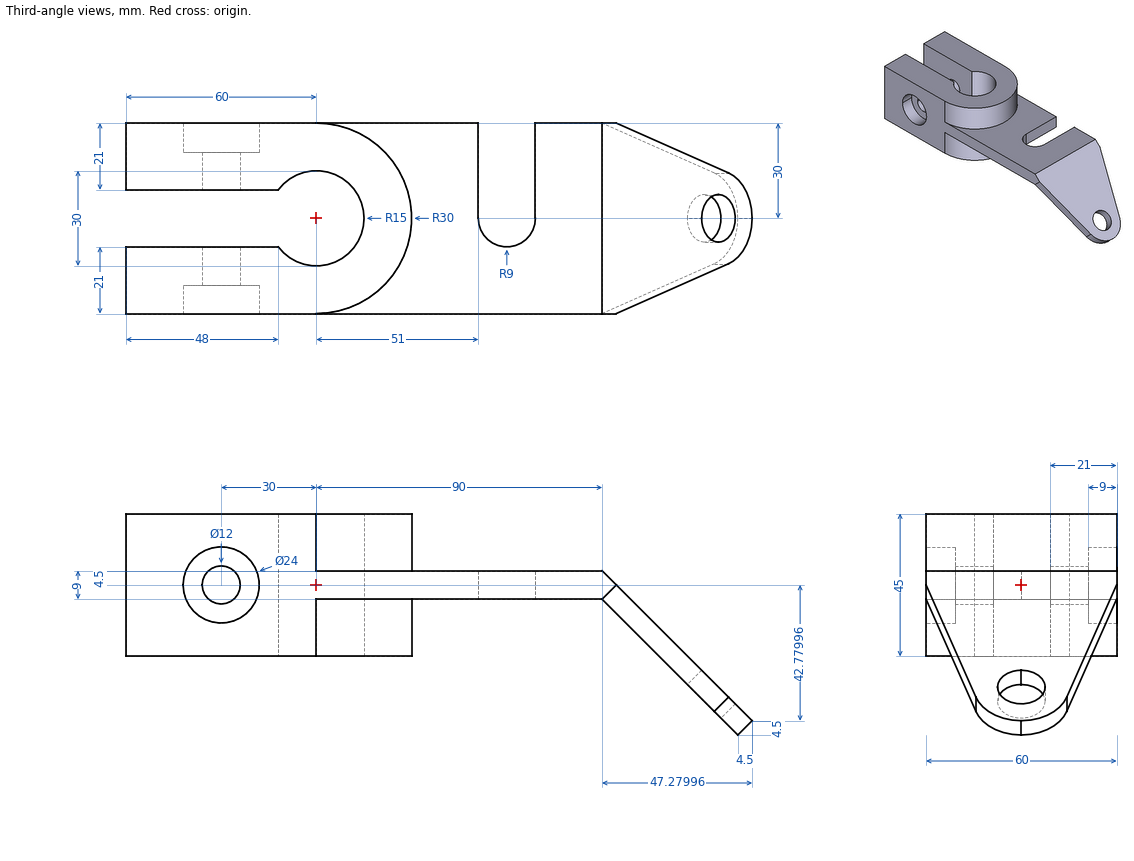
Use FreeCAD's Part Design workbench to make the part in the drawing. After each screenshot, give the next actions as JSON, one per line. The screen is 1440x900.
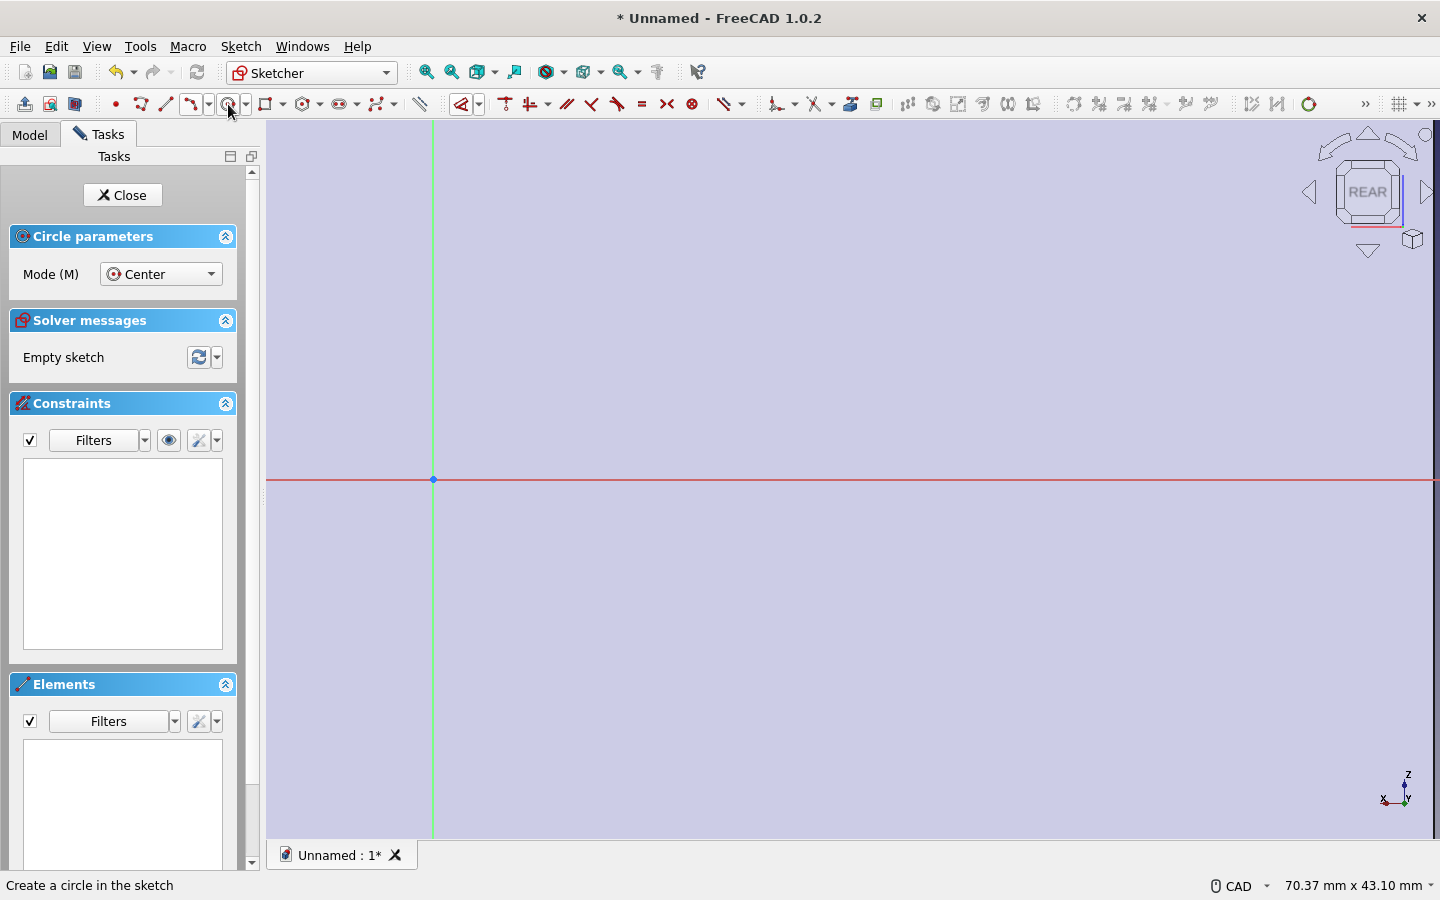
{"action": "left_click", "coordinate": [934, 479]}
{"action": "left_click", "coordinate": [1075, 338]}
{"action": "key", "text": "Escape"}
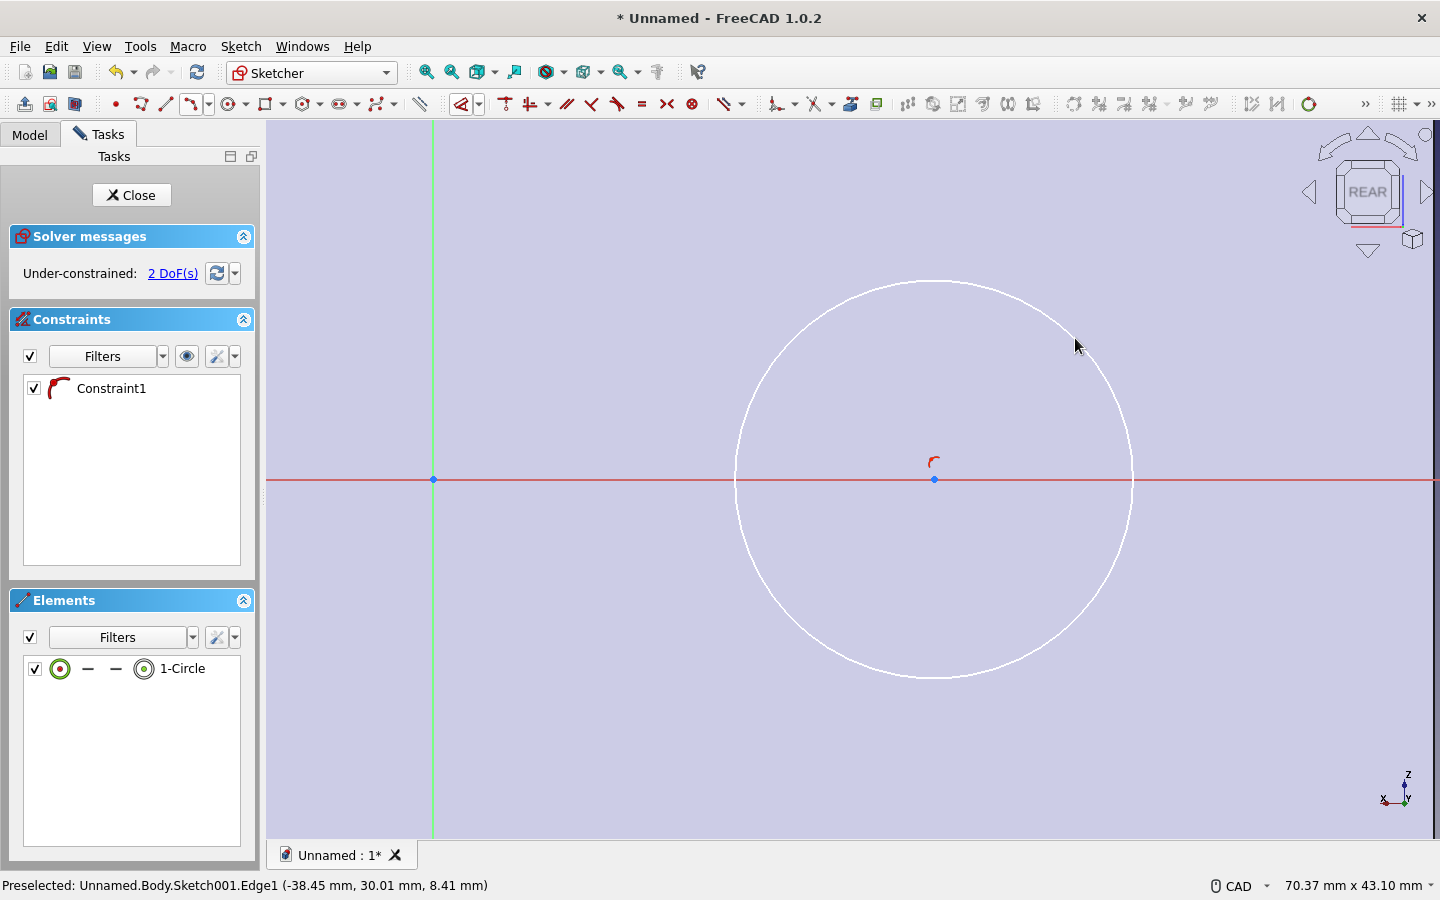
{"action": "left_click", "coordinate": [1074, 338]}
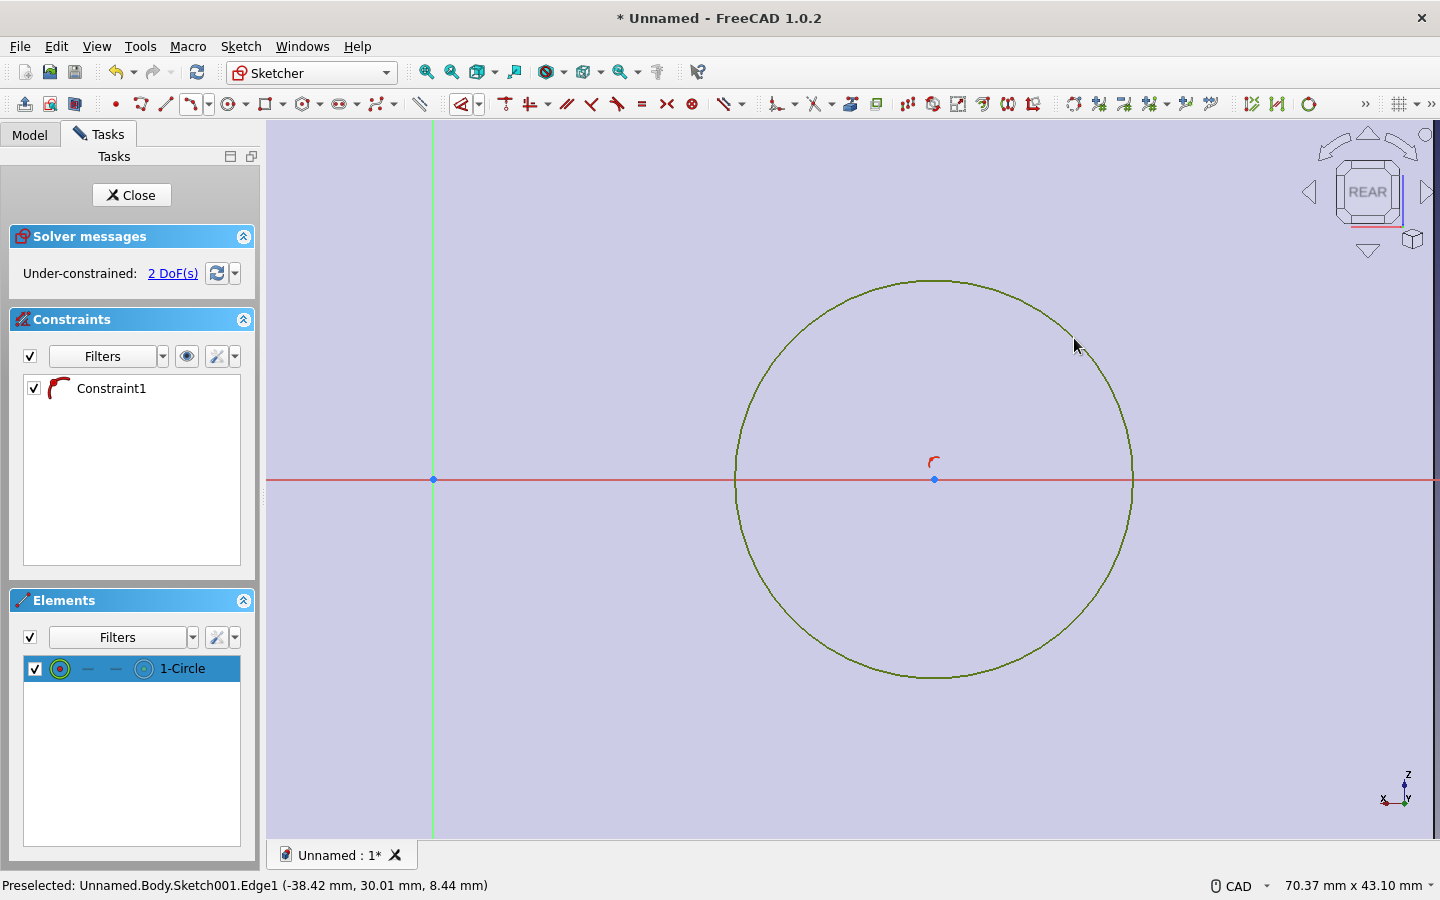
{"action": "key", "text": "k o"}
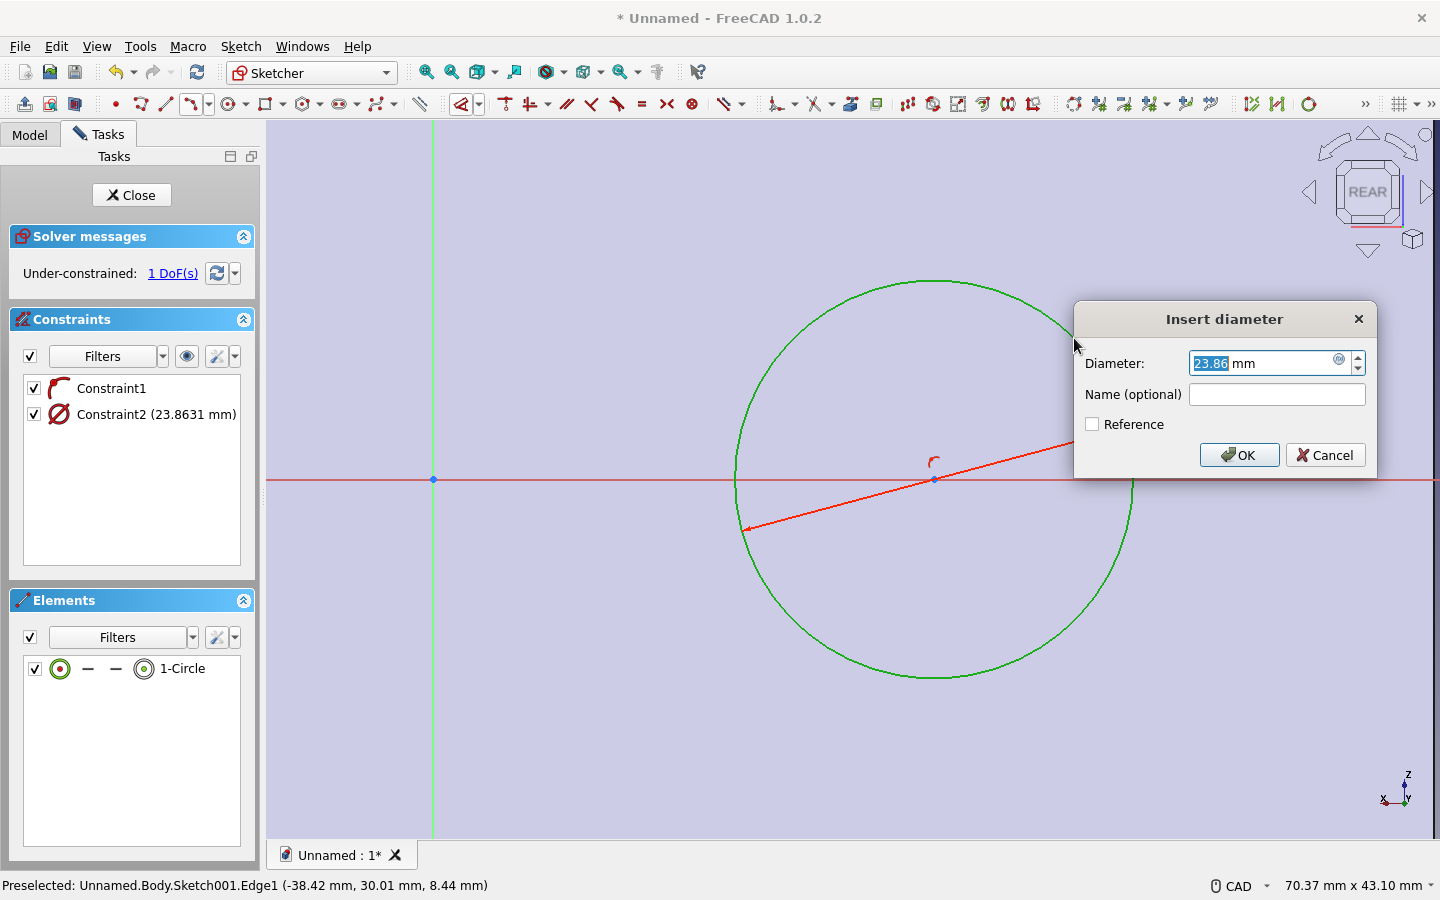
{"action": "type", "text": "24"}
{"action": "key", "text": "Return"}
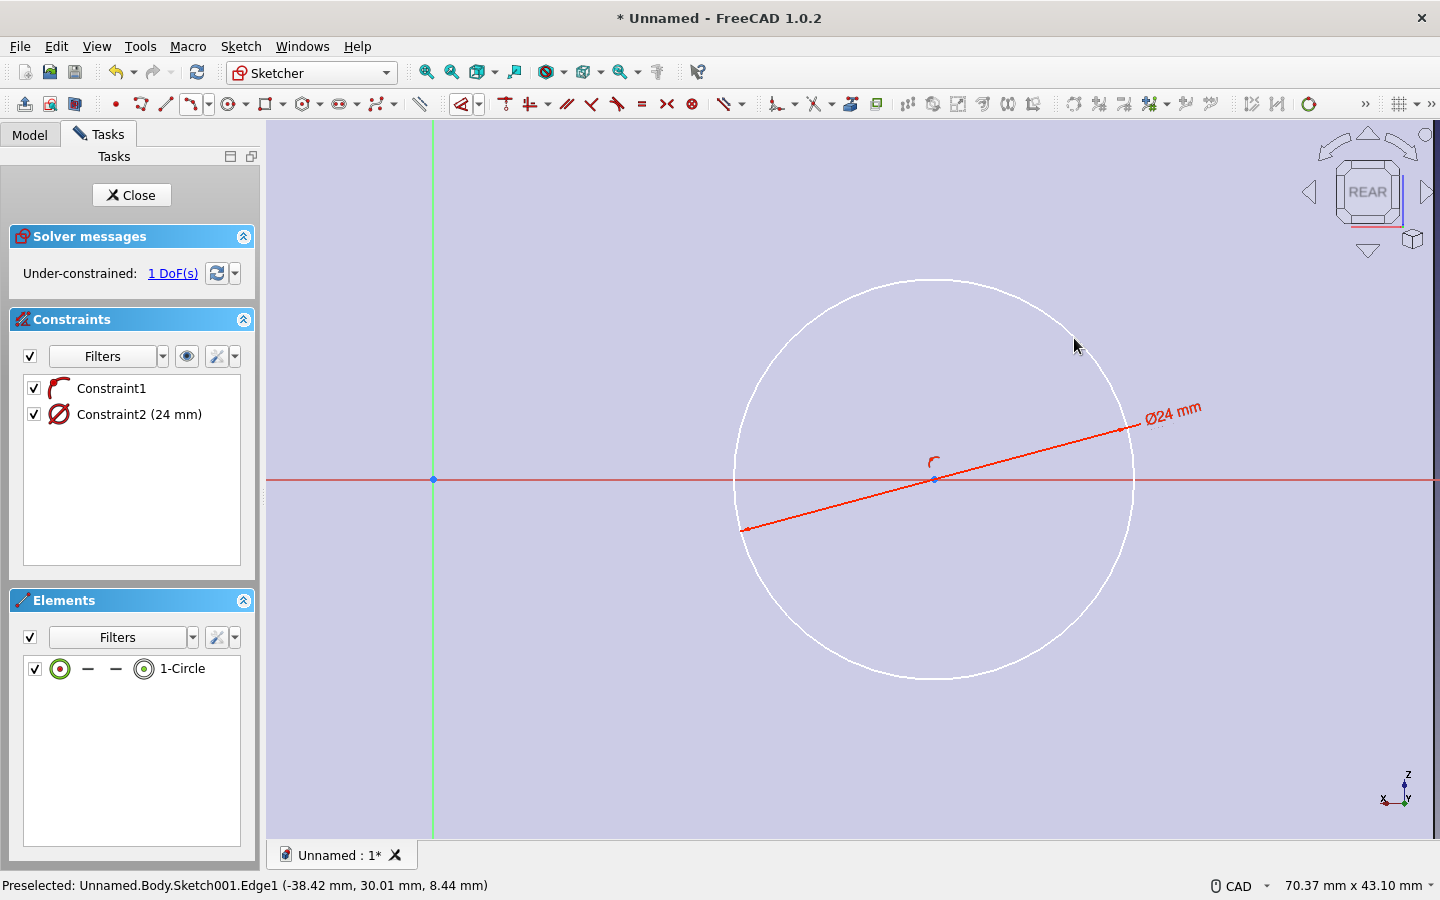
{"action": "left_click", "coordinate": [934, 479]}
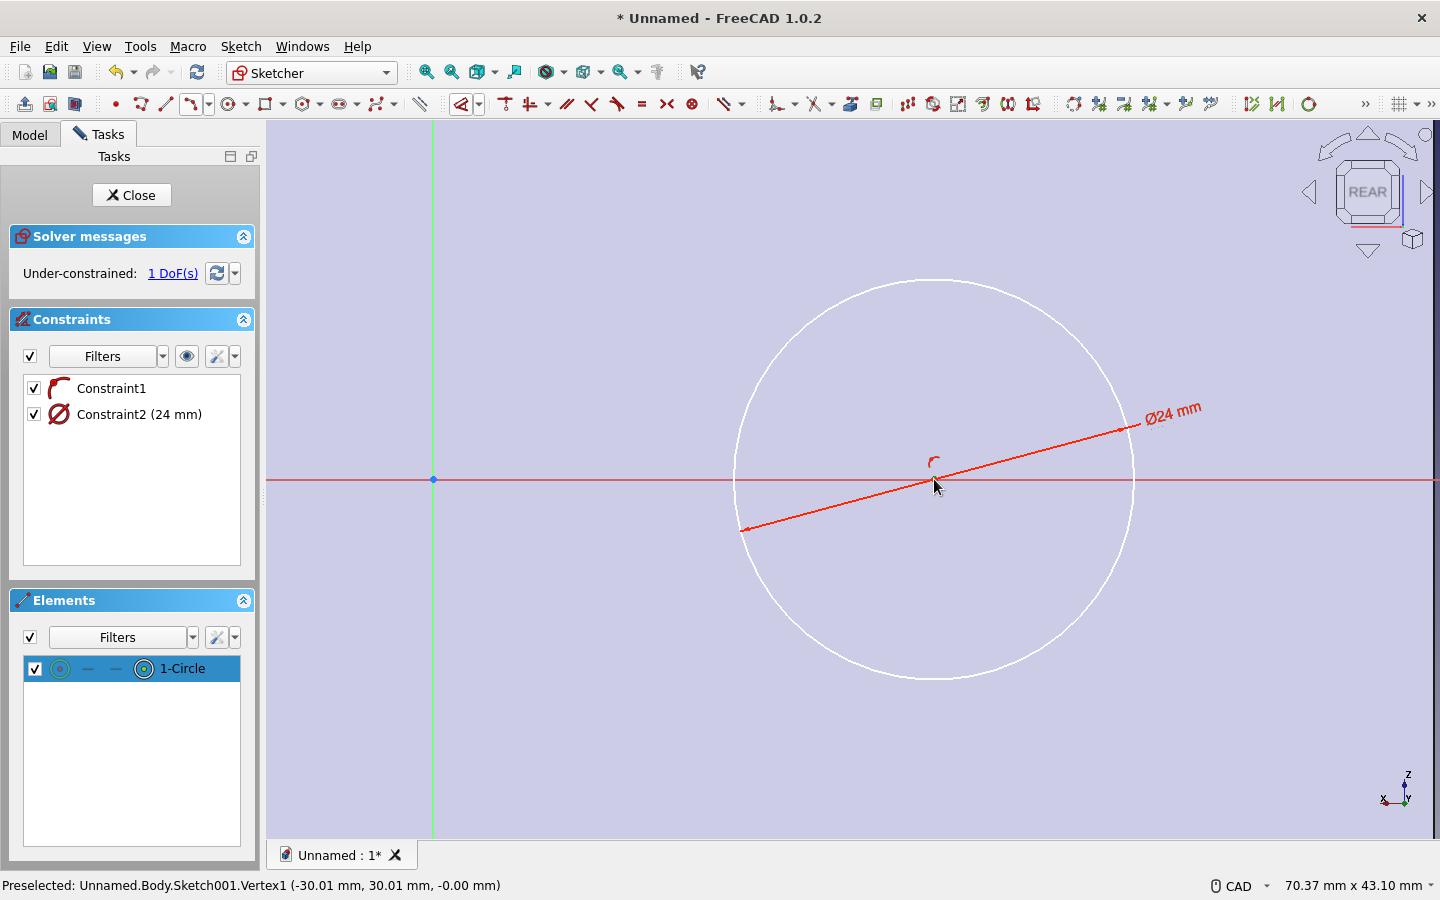
{"action": "key", "text": "l"}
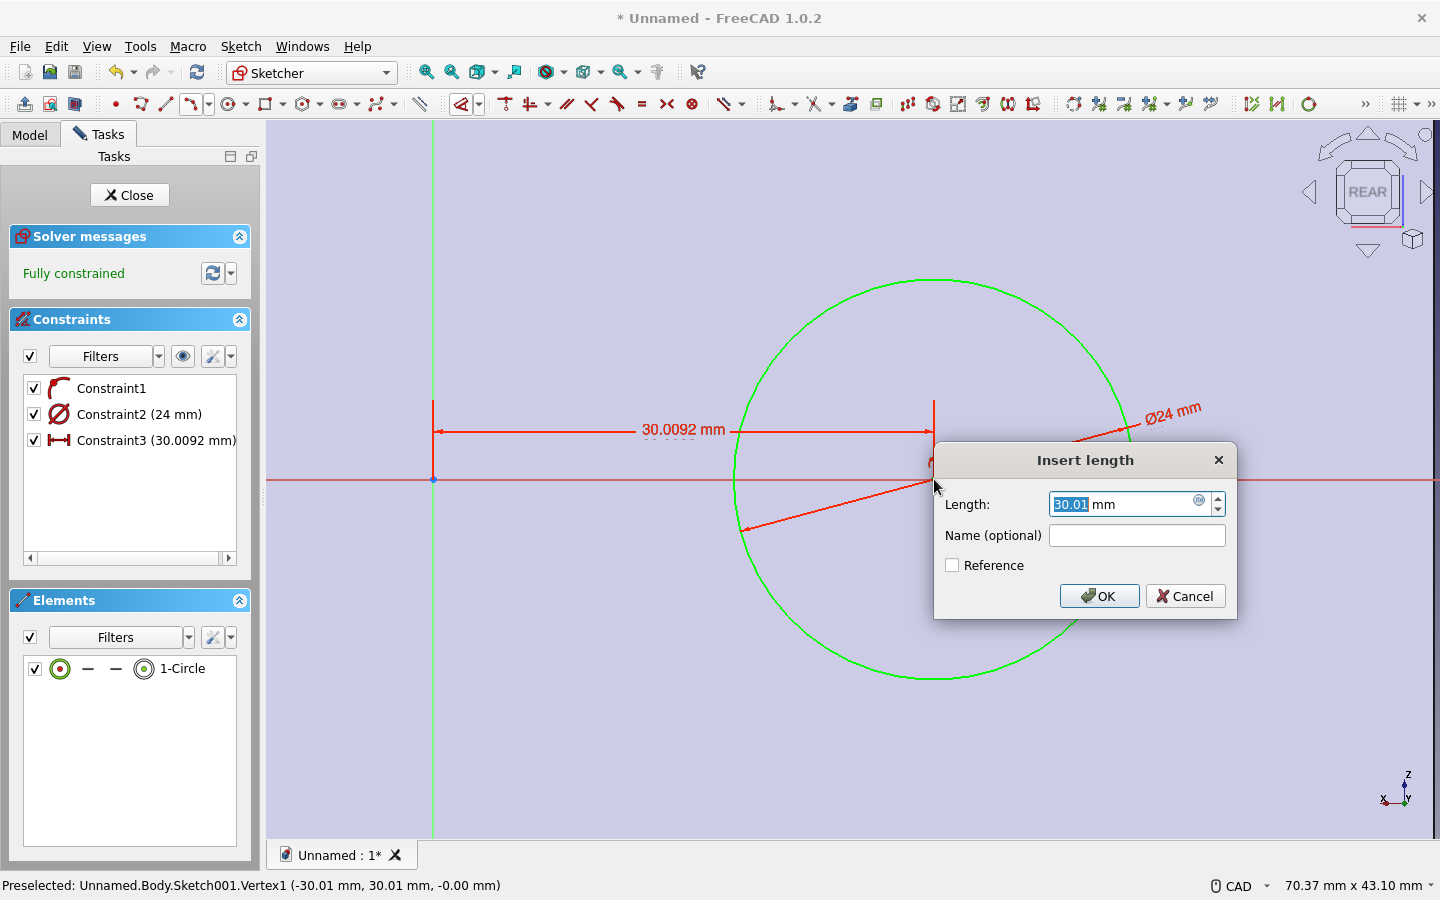
{"action": "type", "text": "30"}
{"action": "key", "text": "Return"}